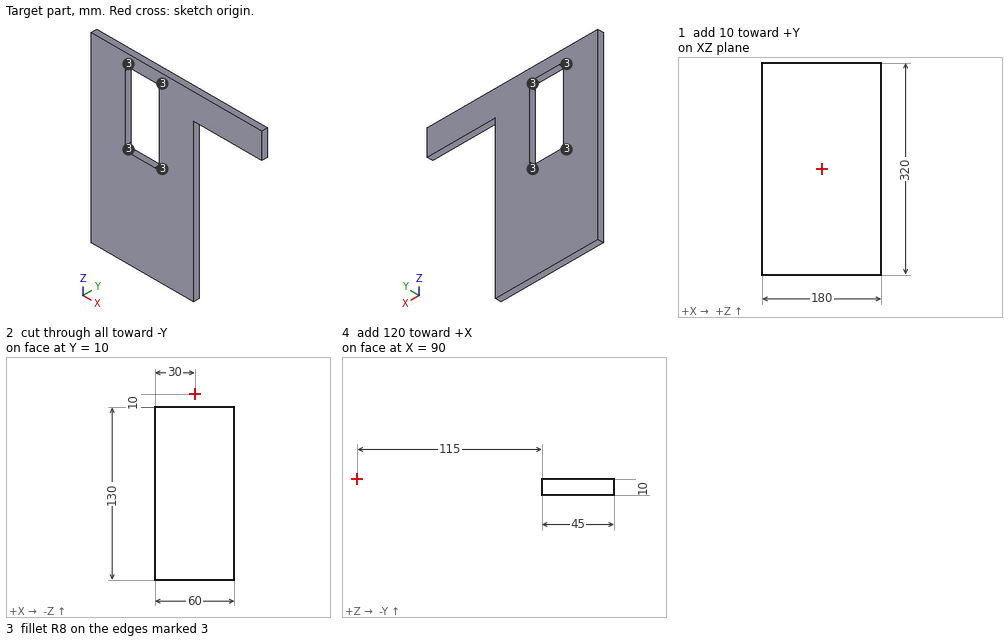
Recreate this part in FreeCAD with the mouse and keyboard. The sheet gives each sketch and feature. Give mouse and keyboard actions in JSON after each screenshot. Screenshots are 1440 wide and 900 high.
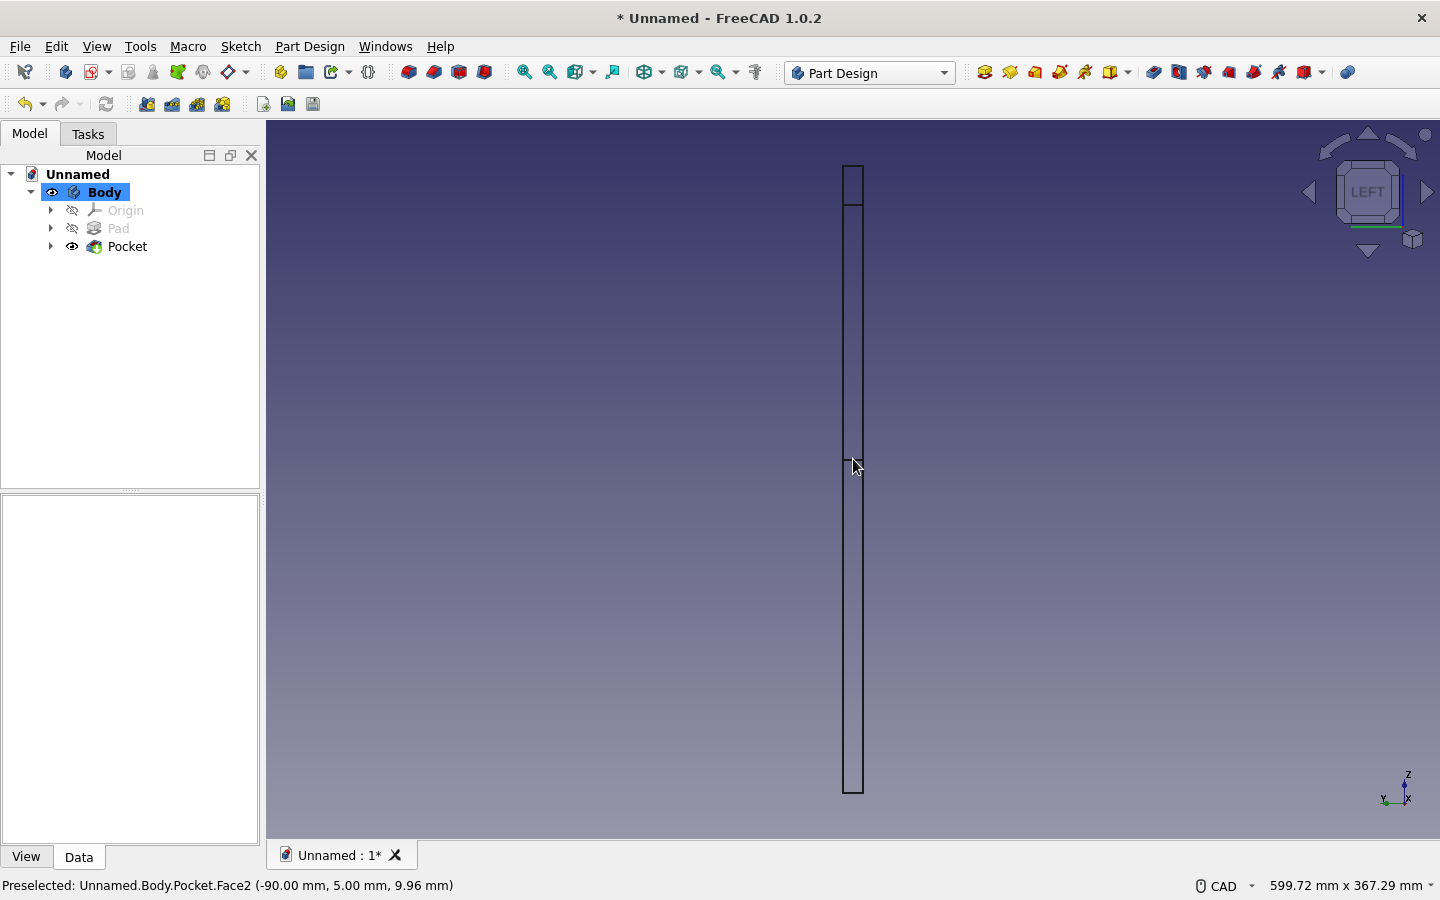
{"action": "key", "text": "0"}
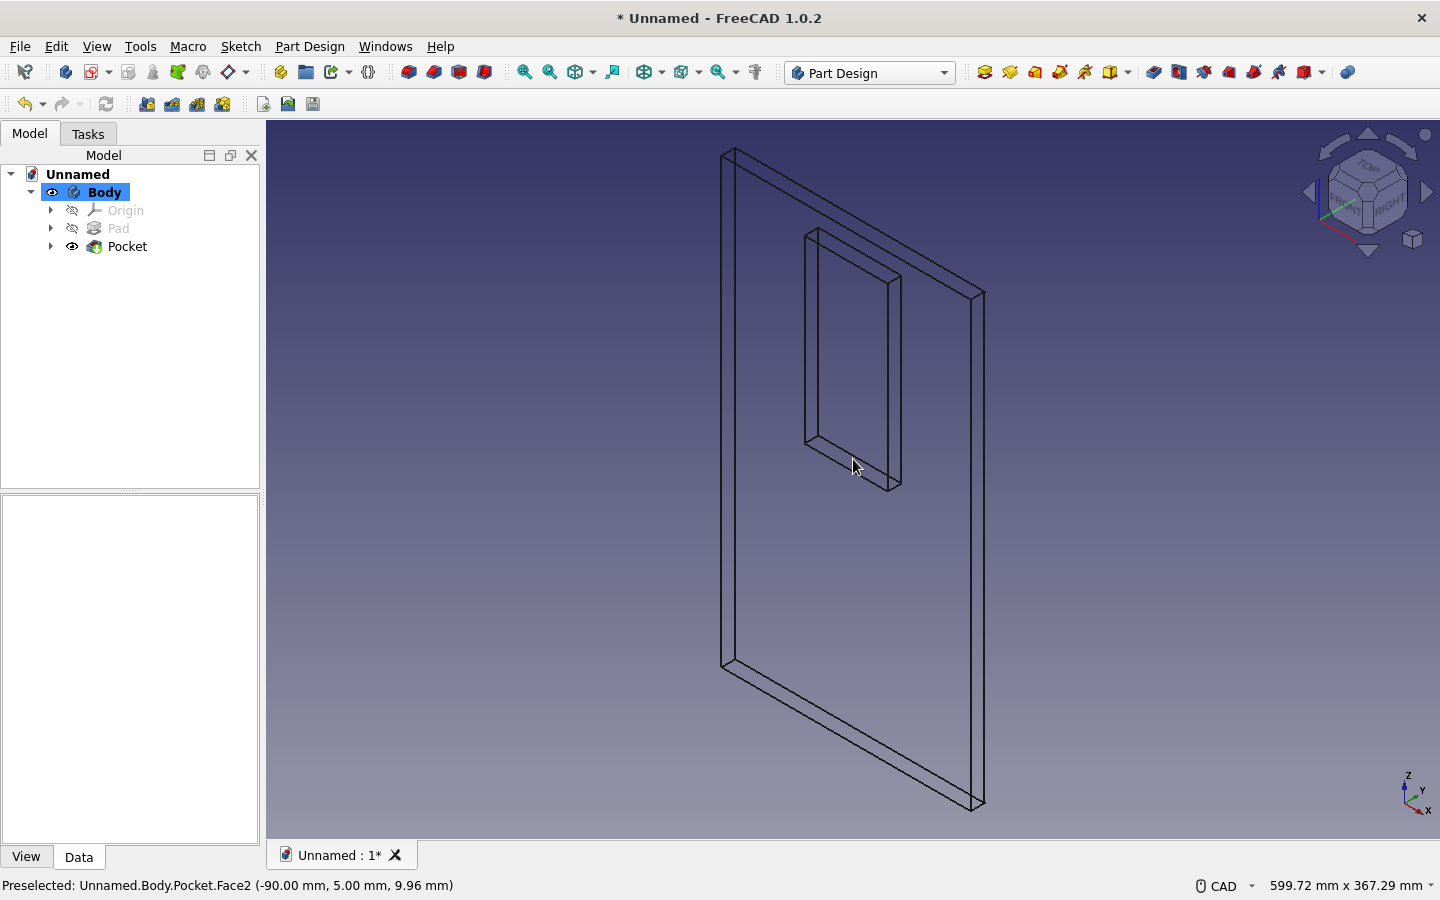
{"action": "left_click", "coordinate": [895, 486]}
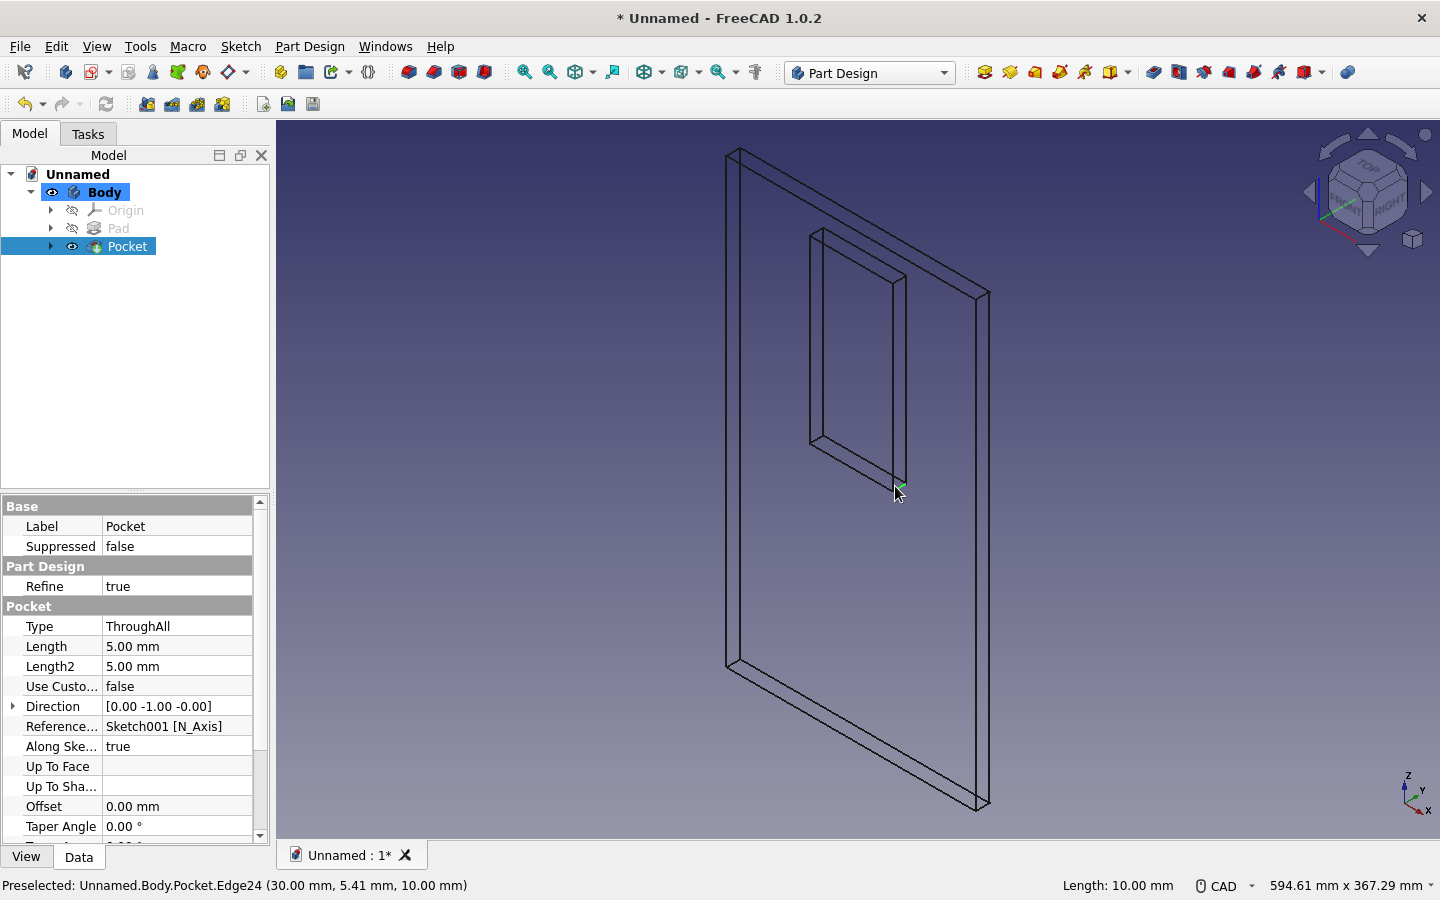
{"action": "left_click", "coordinate": [900, 279], "text": "ctrl"}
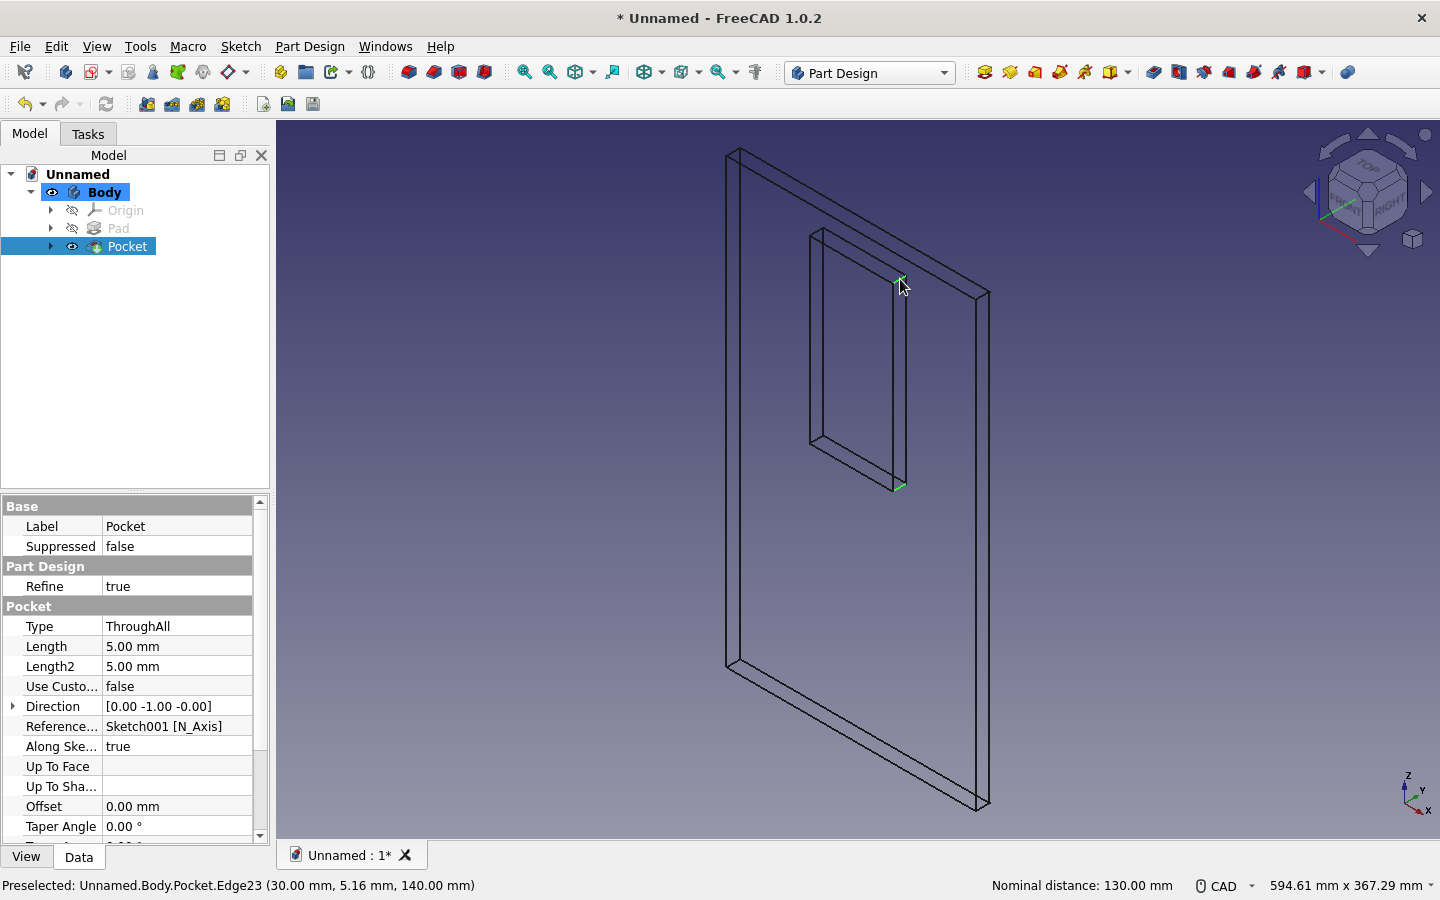
{"action": "left_click", "coordinate": [816, 231], "text": "ctrl"}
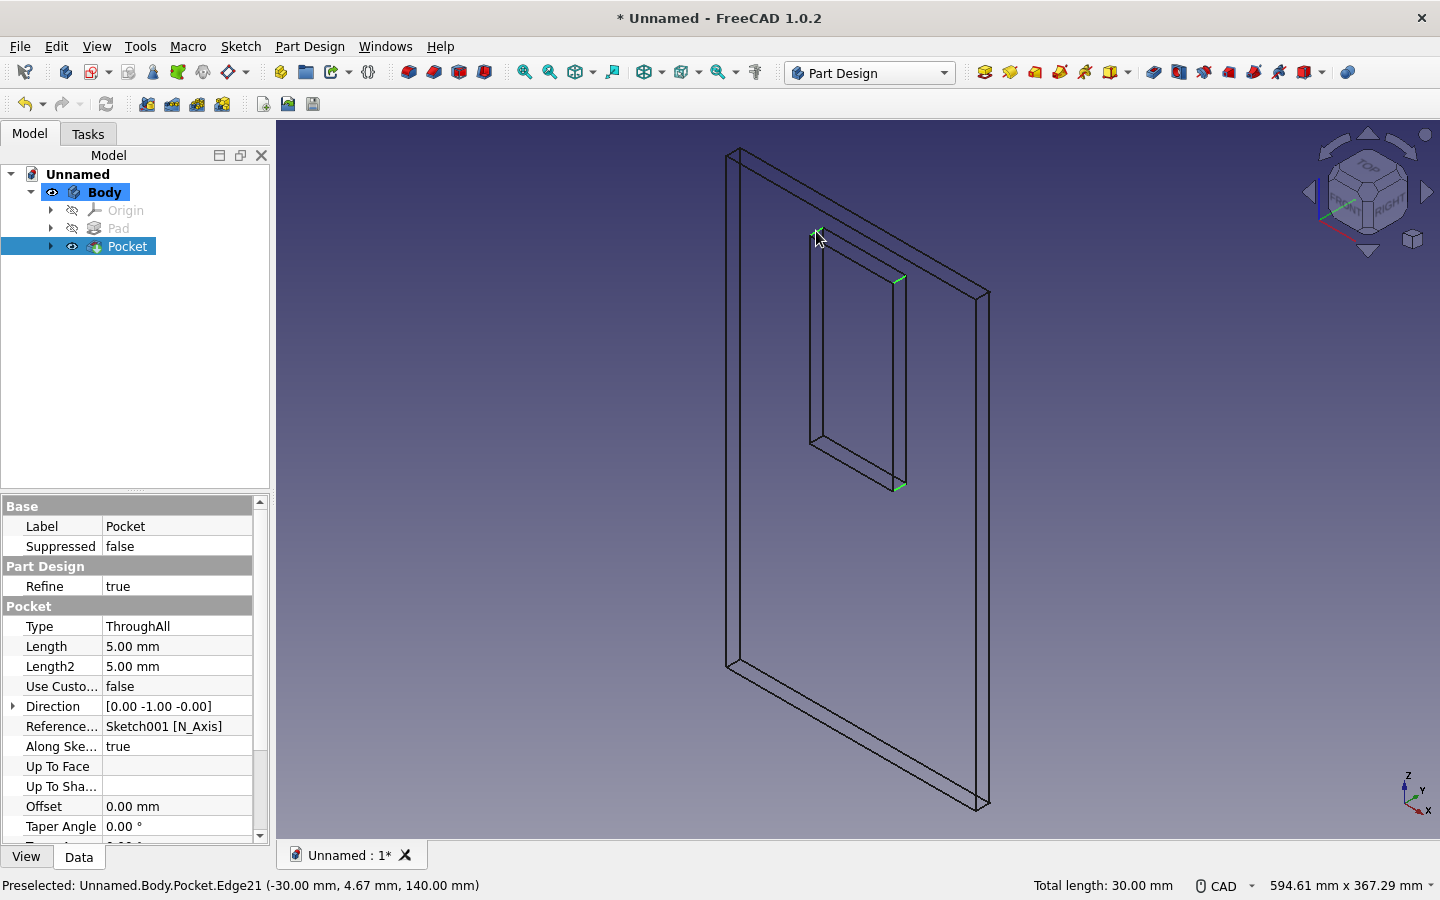
{"action": "left_click", "coordinate": [818, 438], "text": "ctrl"}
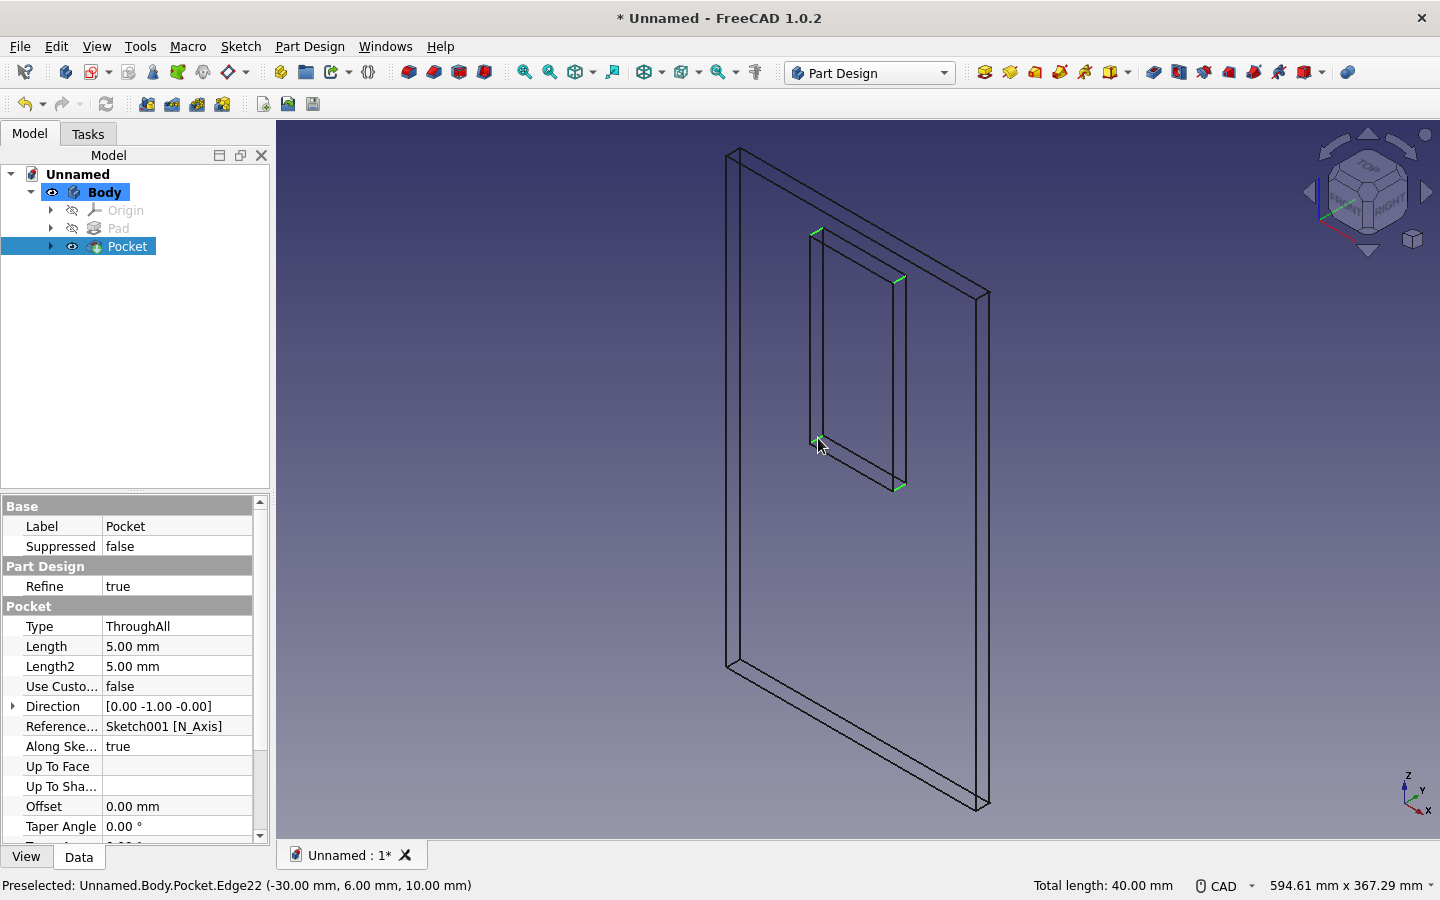
{"action": "key", "text": "v 1"}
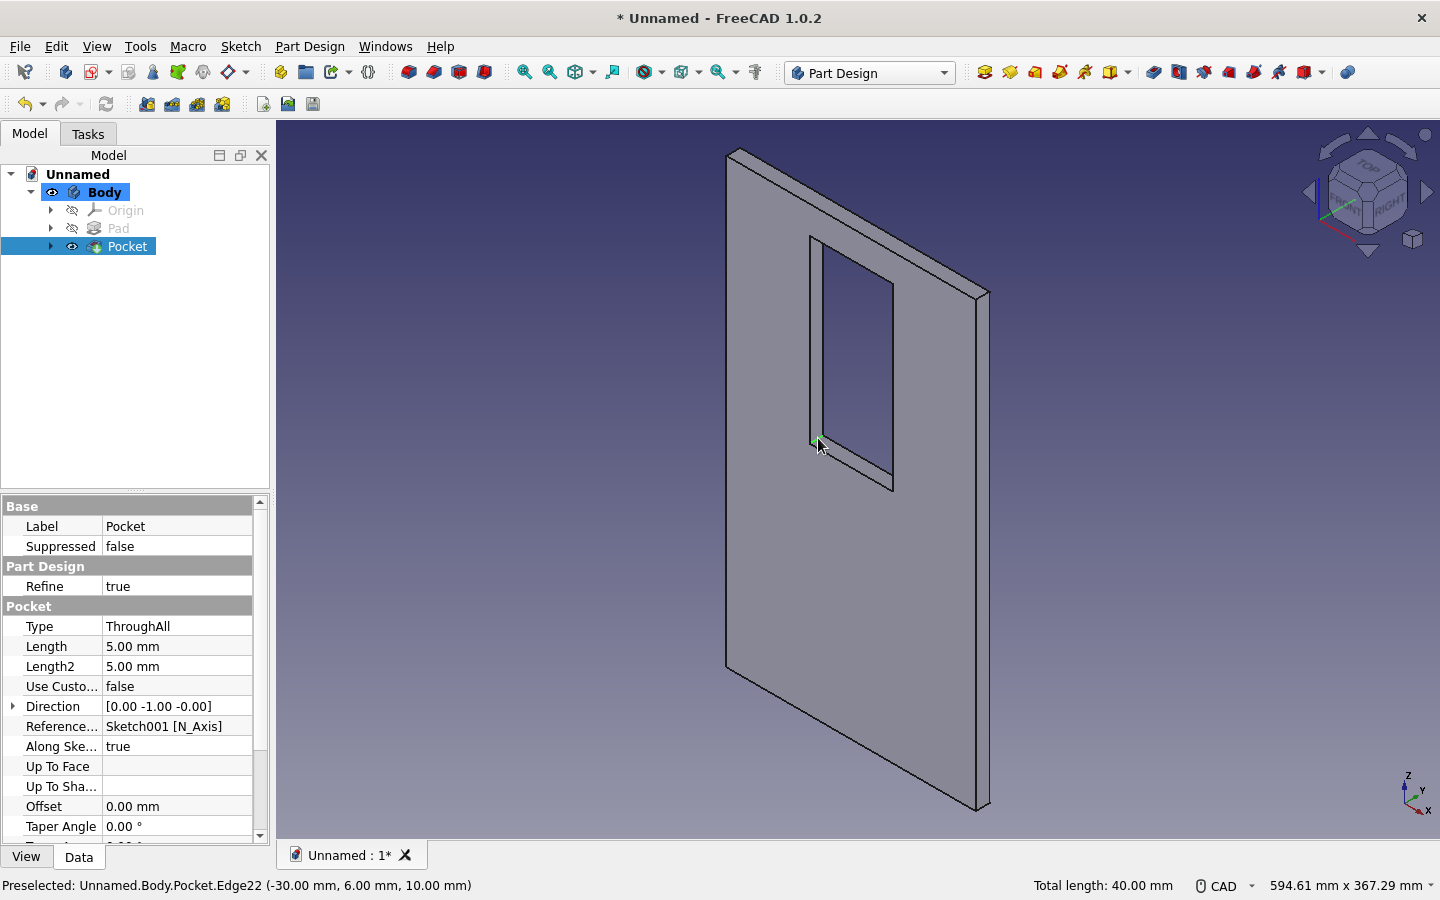
{"action": "left_click", "coordinate": [409, 72]}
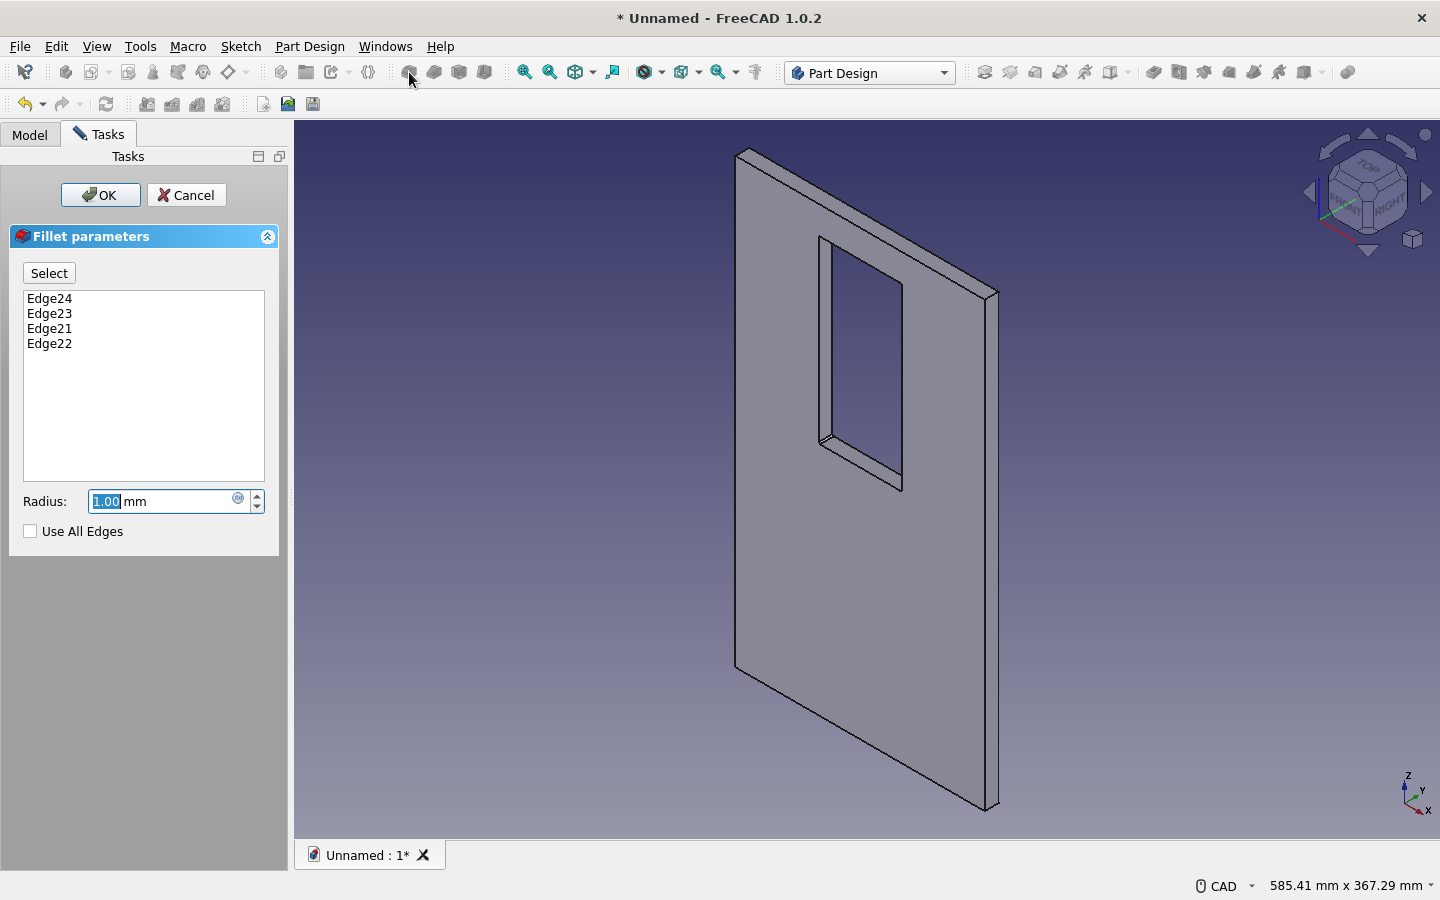
{"action": "type", "text": "8"}
{"action": "key", "text": "Tab"}